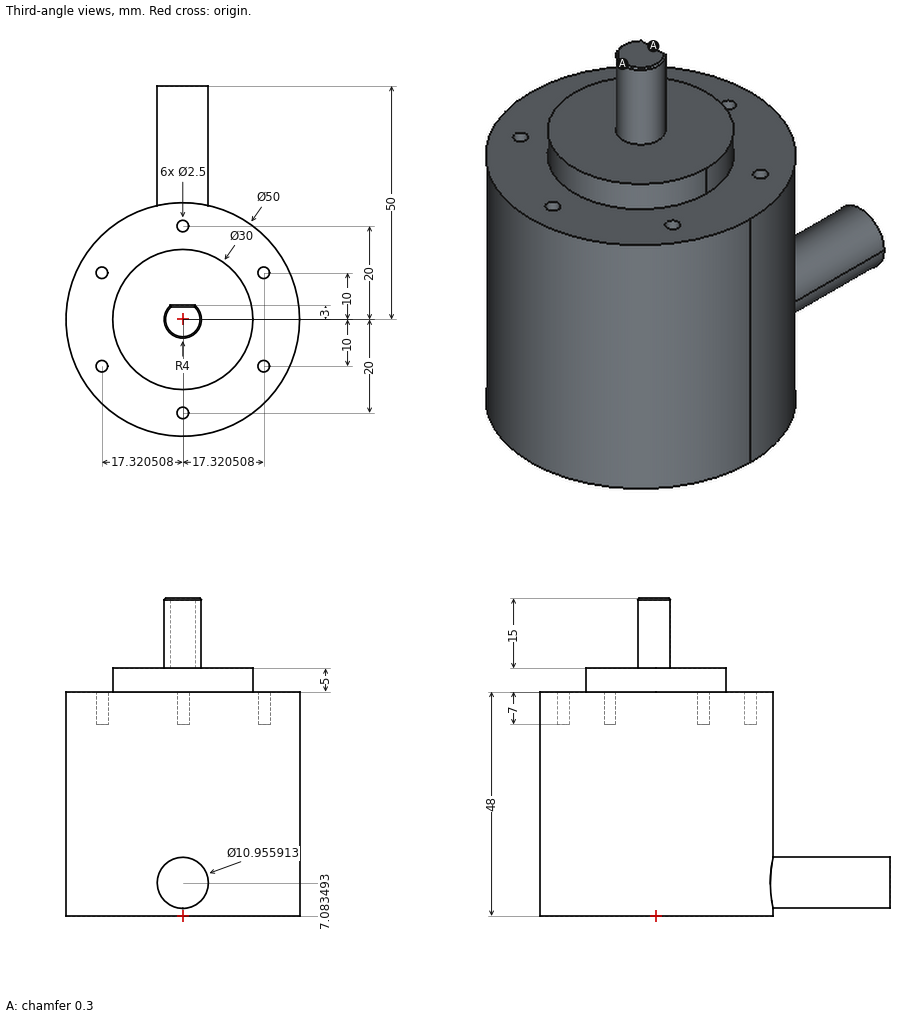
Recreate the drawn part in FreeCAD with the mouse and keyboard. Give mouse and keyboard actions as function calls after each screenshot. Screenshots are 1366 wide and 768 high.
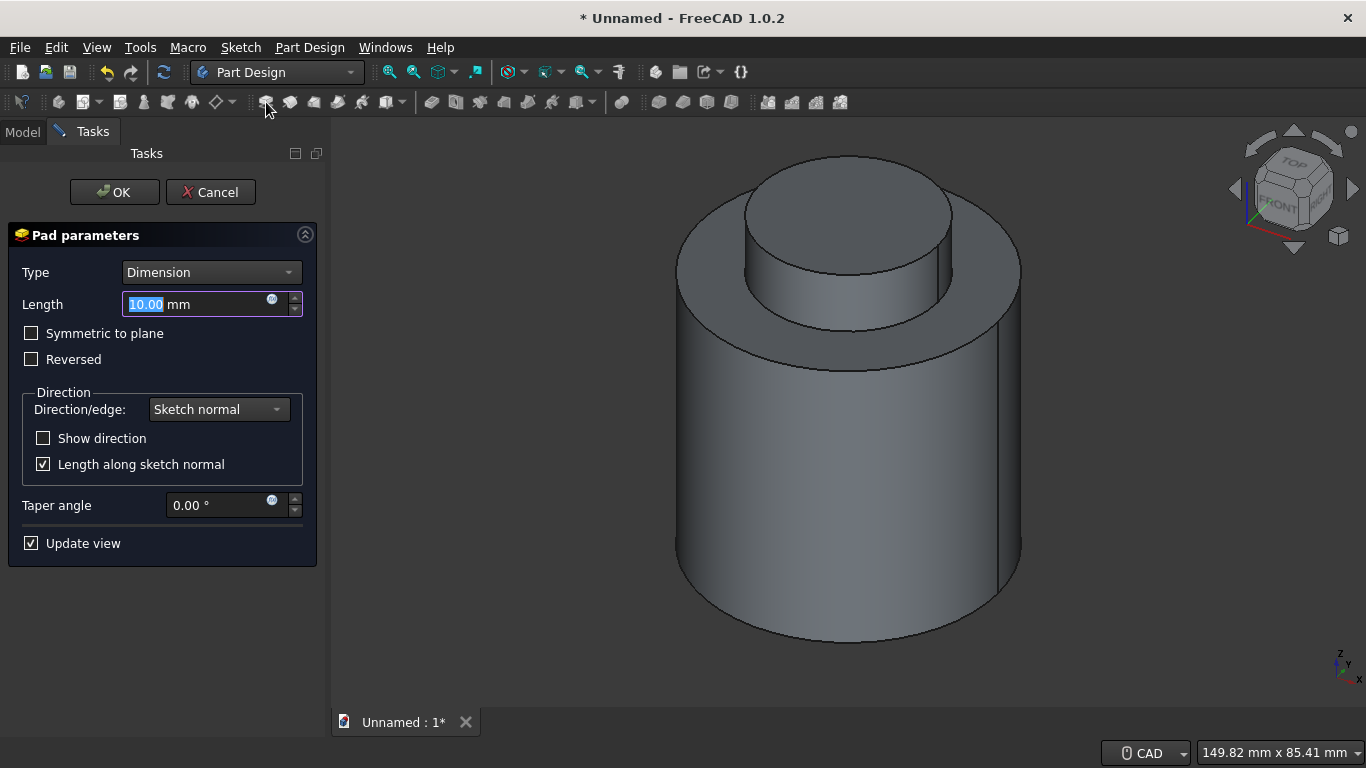
text(5)
key(Tab)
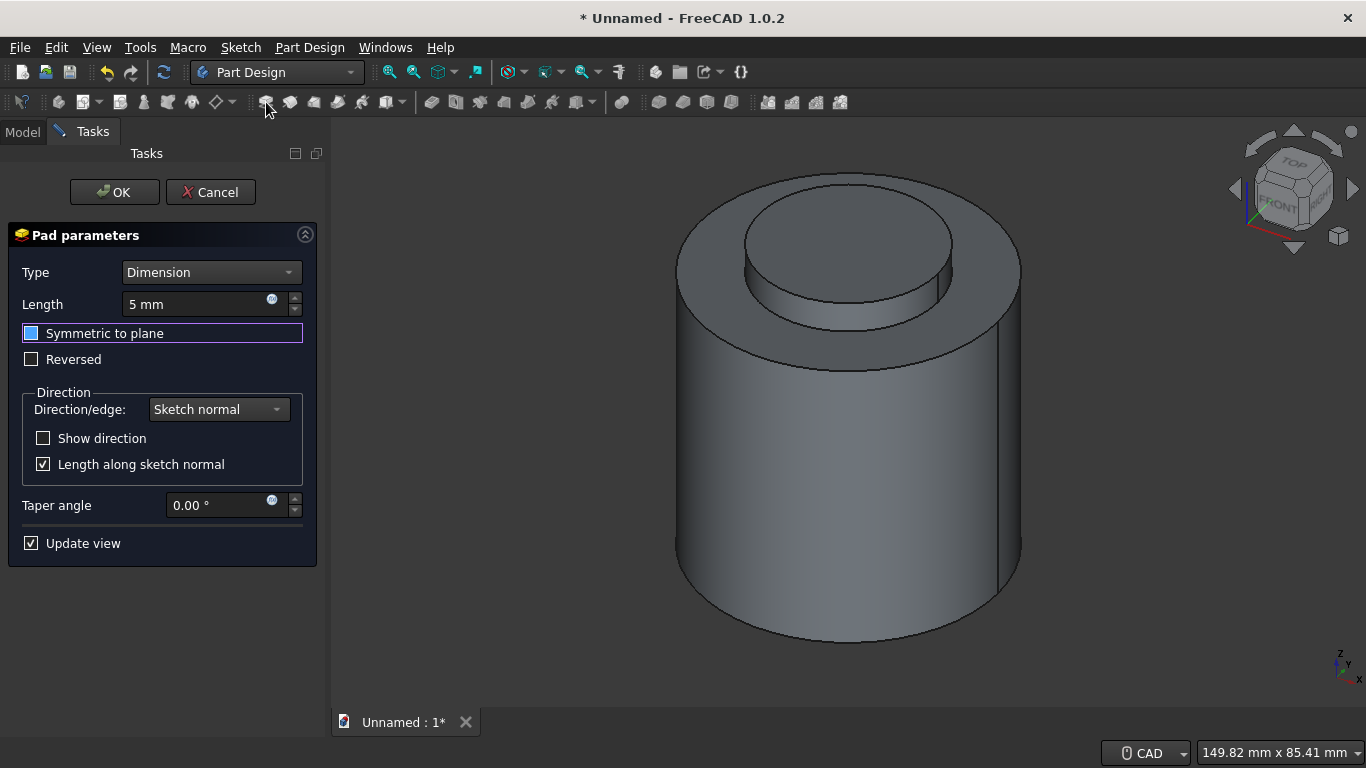
click(115, 192)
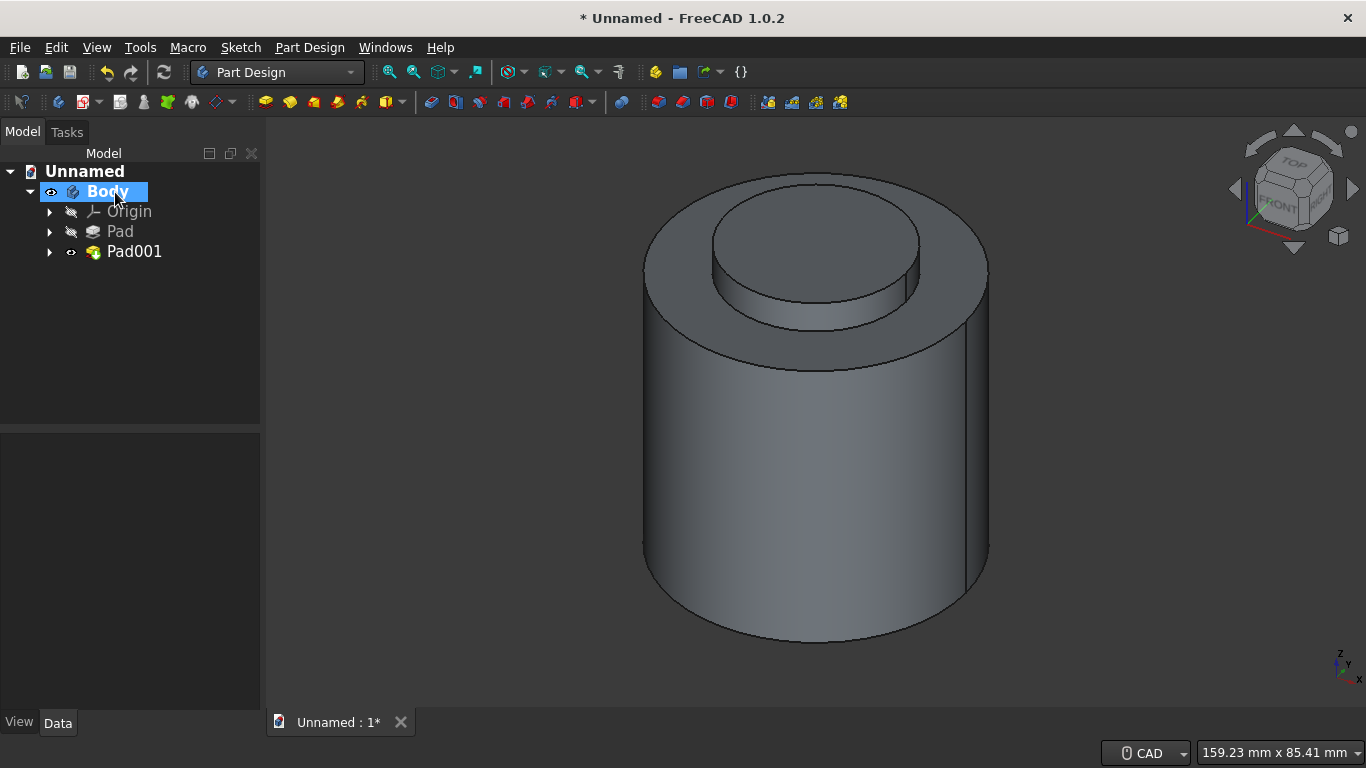
click(390, 72)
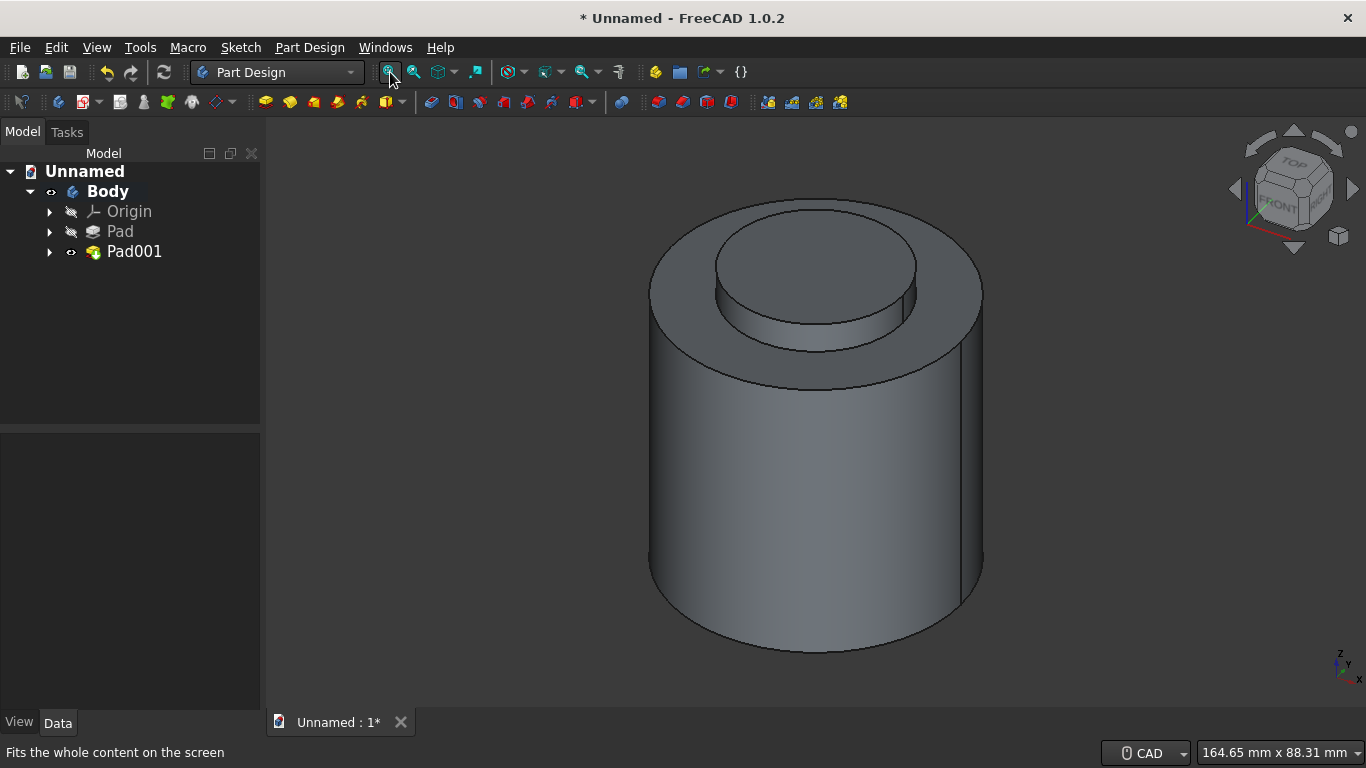
click(816, 266)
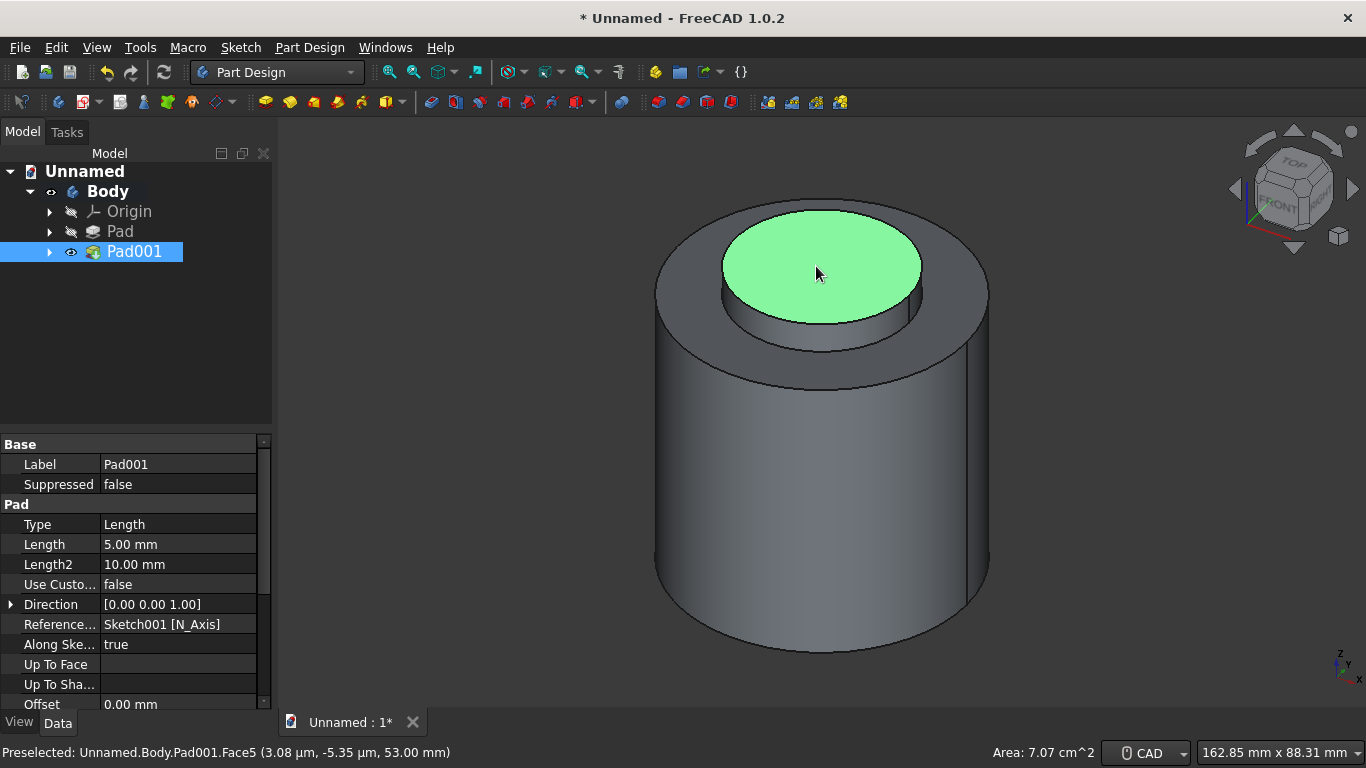
click(84, 102)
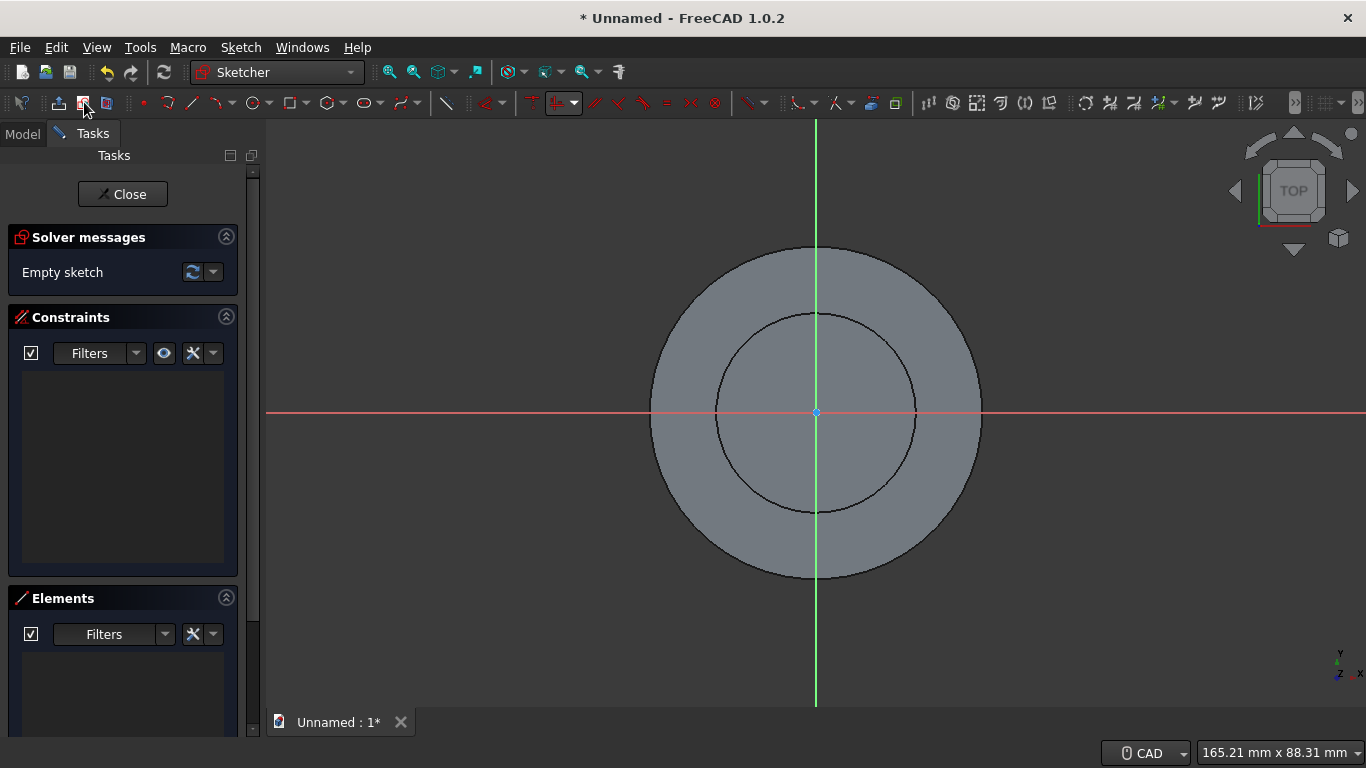
scroll(827, 417, up, 10)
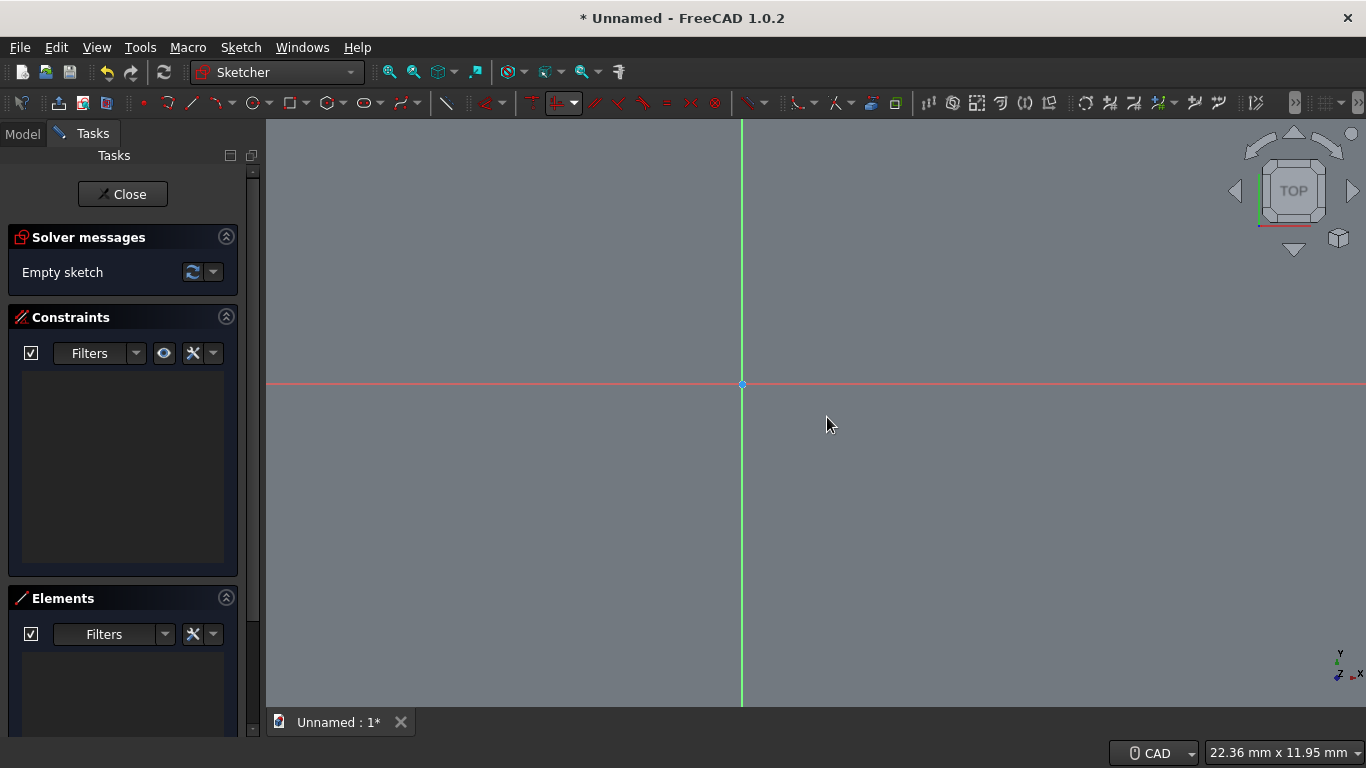
click(192, 104)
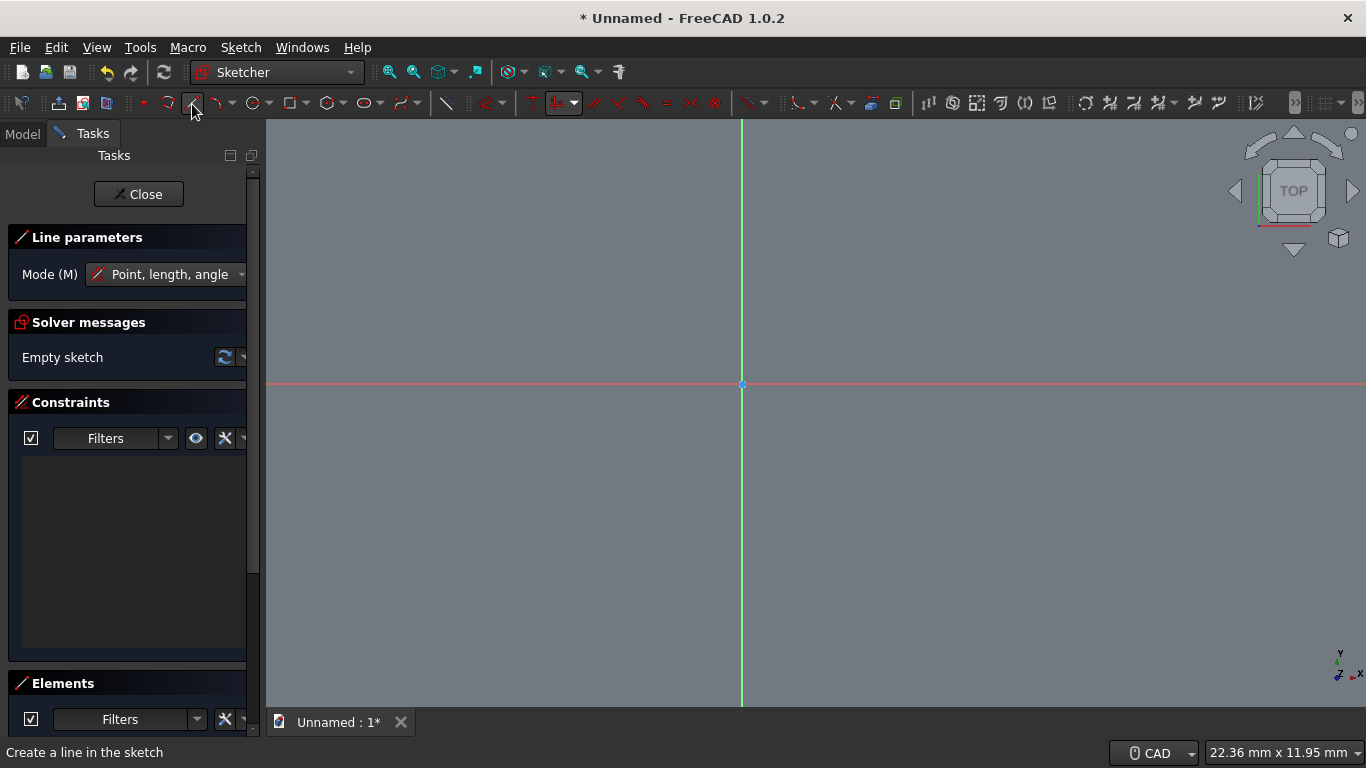
click(873, 237)
click(612, 237)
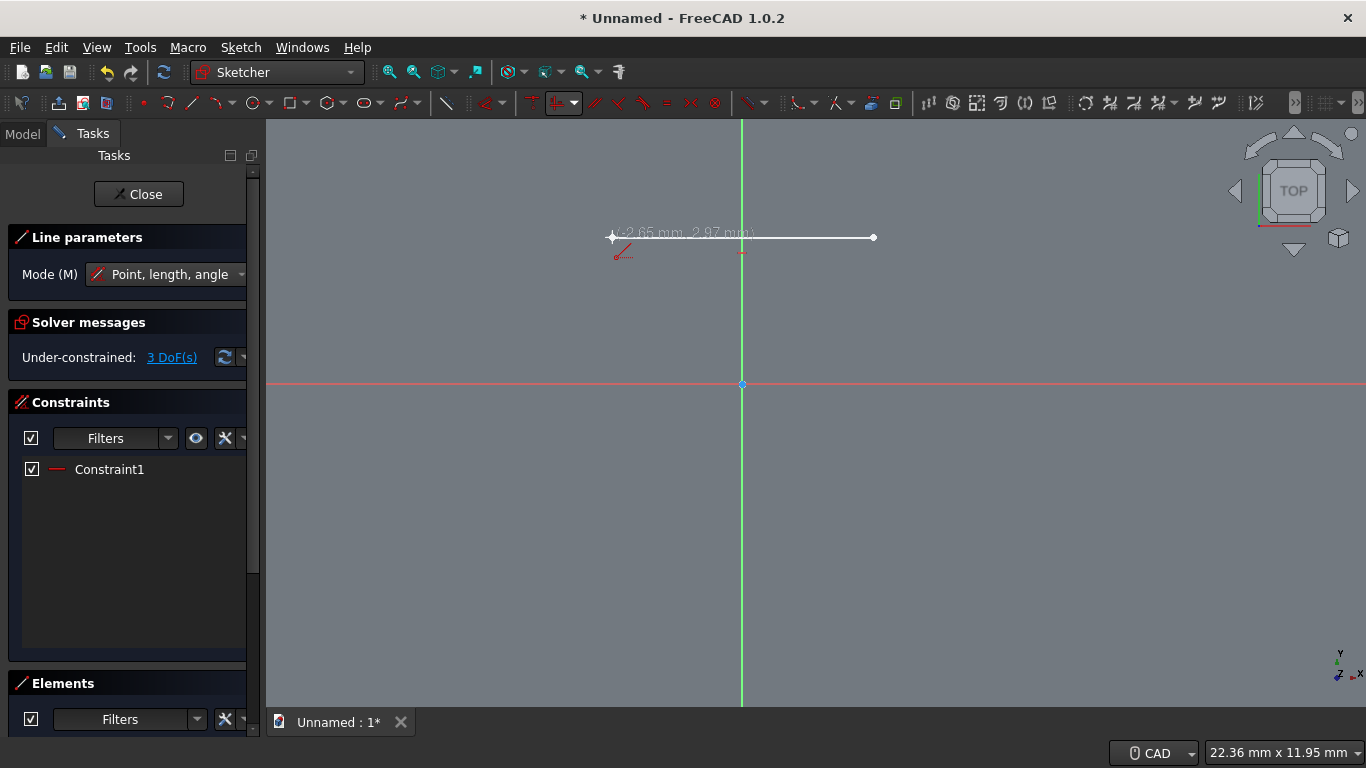
click(216, 104)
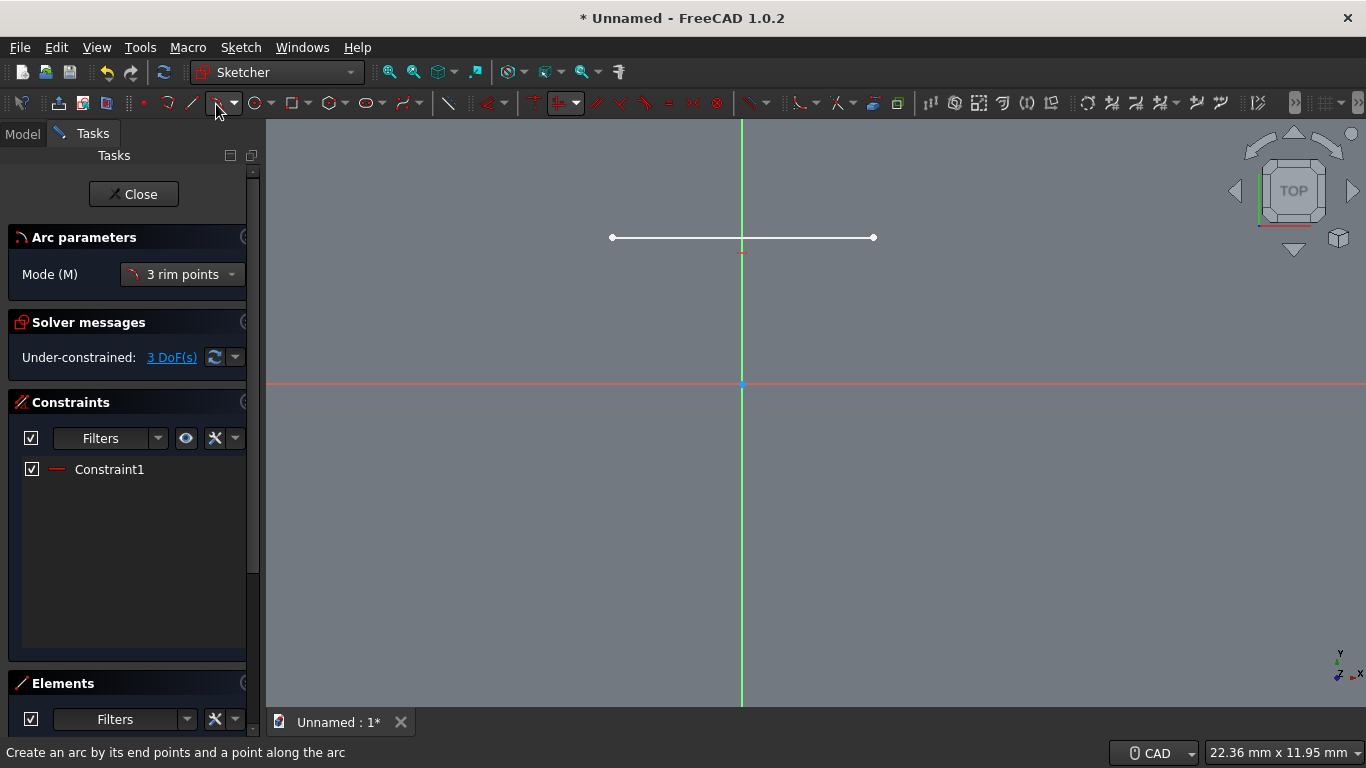
click(612, 238)
click(873, 238)
click(651, 558)
key(Escape)